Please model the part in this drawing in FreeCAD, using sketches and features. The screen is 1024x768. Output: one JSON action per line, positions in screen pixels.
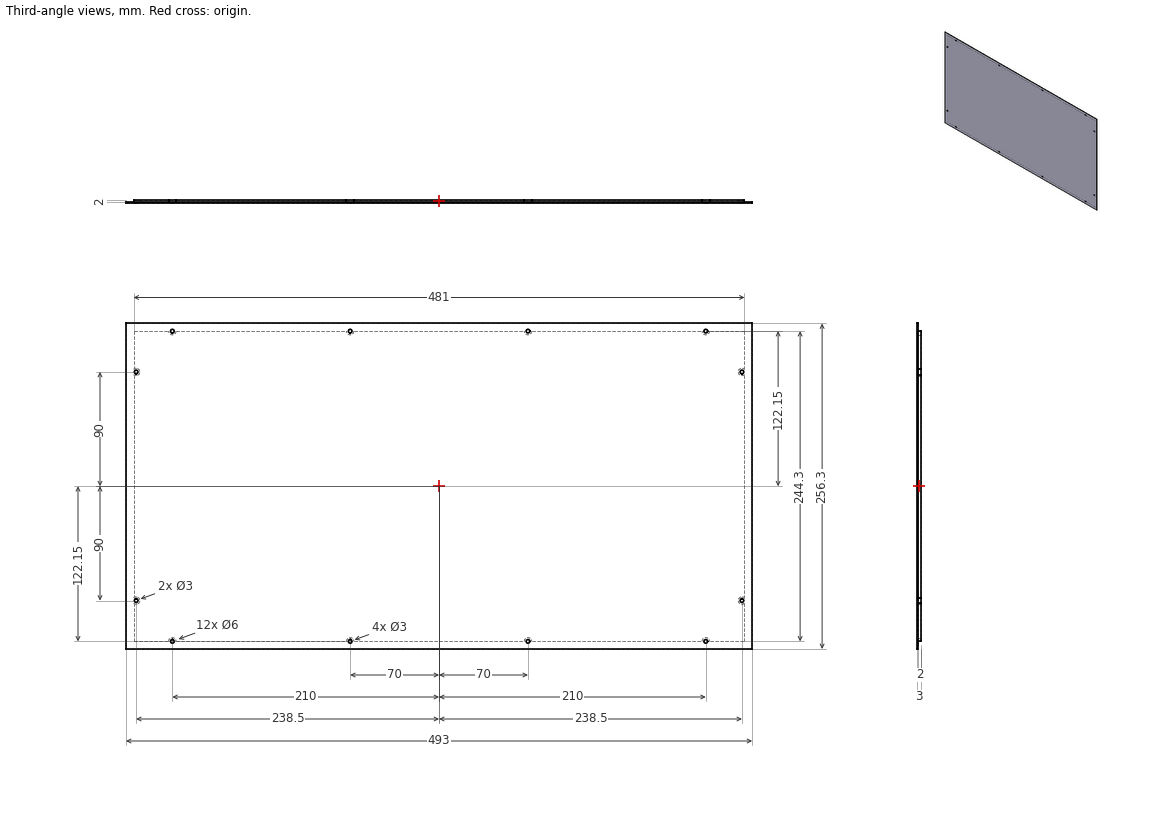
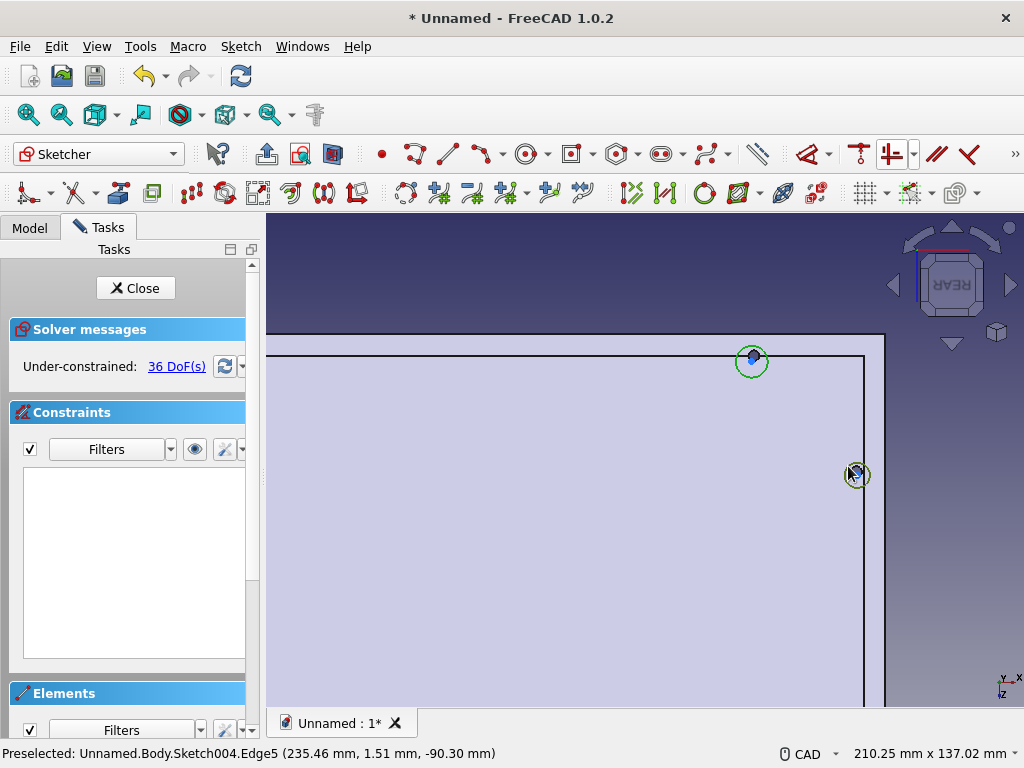
{"action": "scroll", "coordinate": [766, 350], "scroll_direction": "down", "scroll_amount": 7}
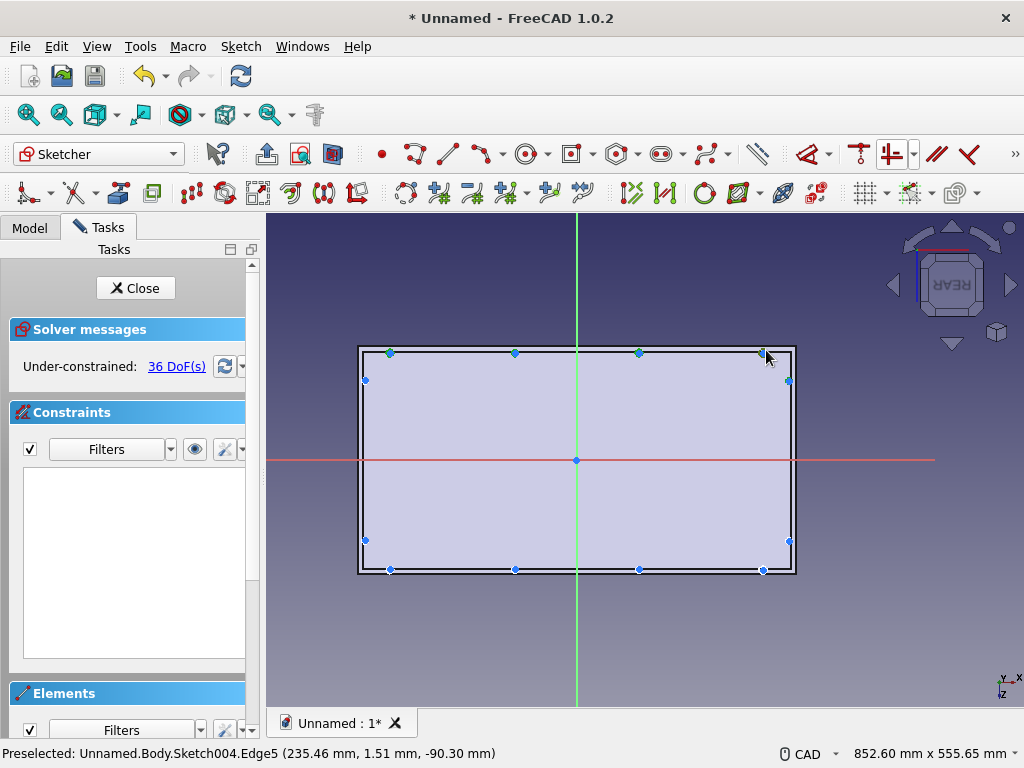
{"action": "scroll", "coordinate": [791, 539], "scroll_direction": "up", "scroll_amount": 8}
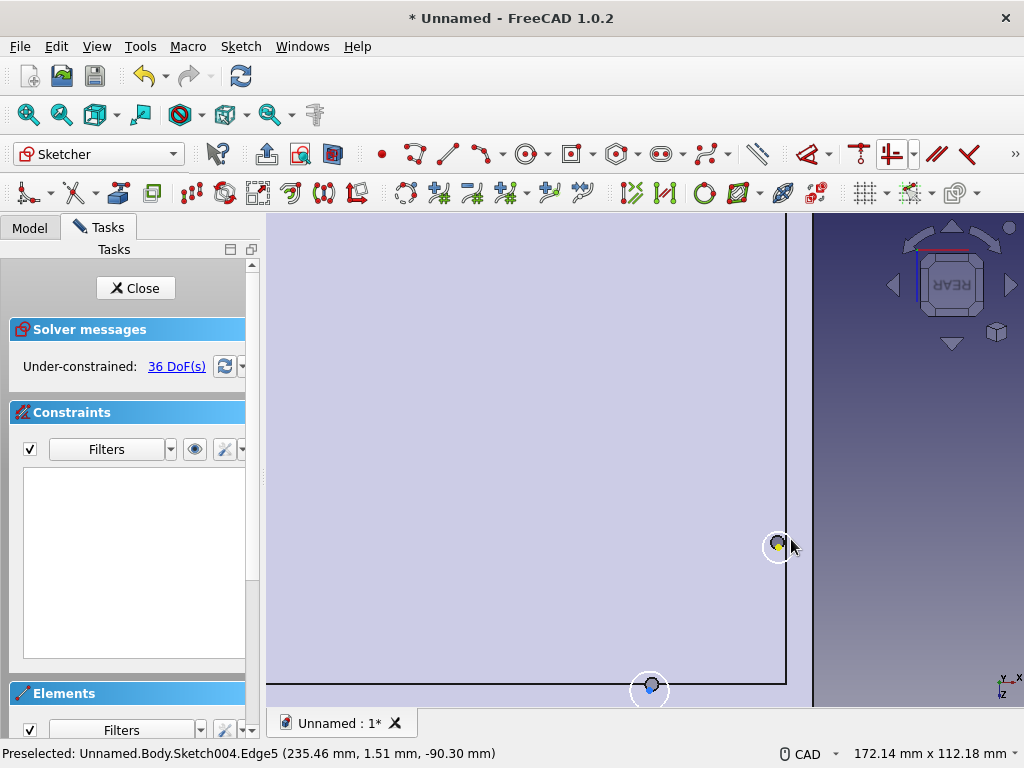
{"action": "left_click", "coordinate": [789, 536]}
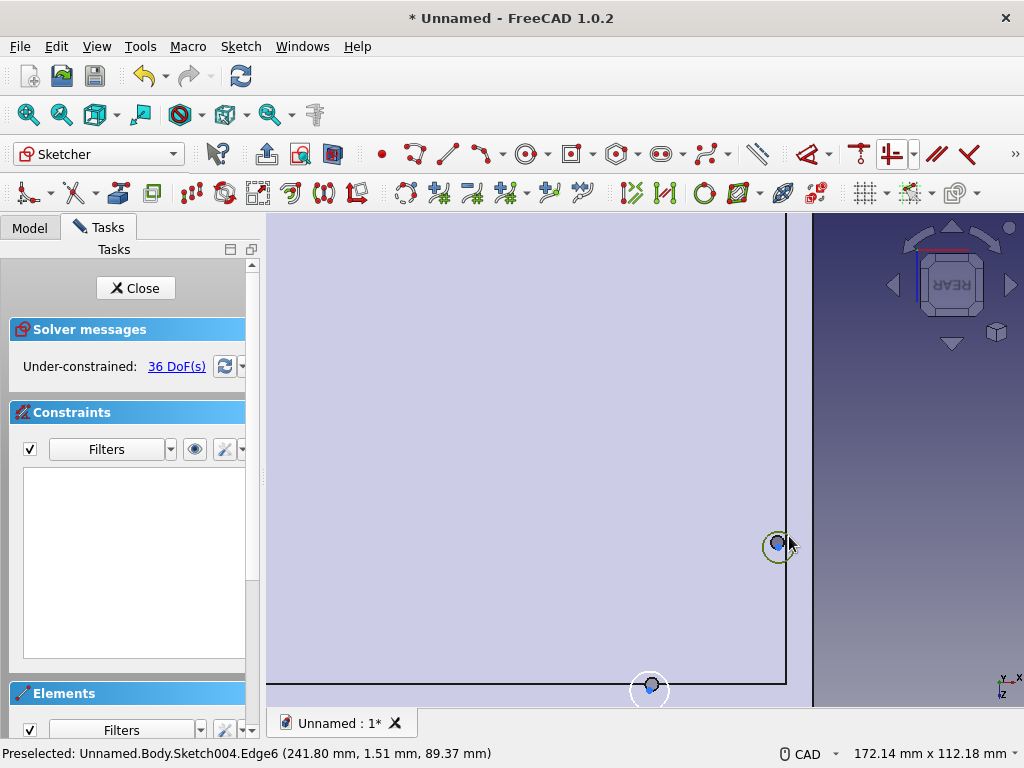
{"action": "left_click", "coordinate": [663, 677]}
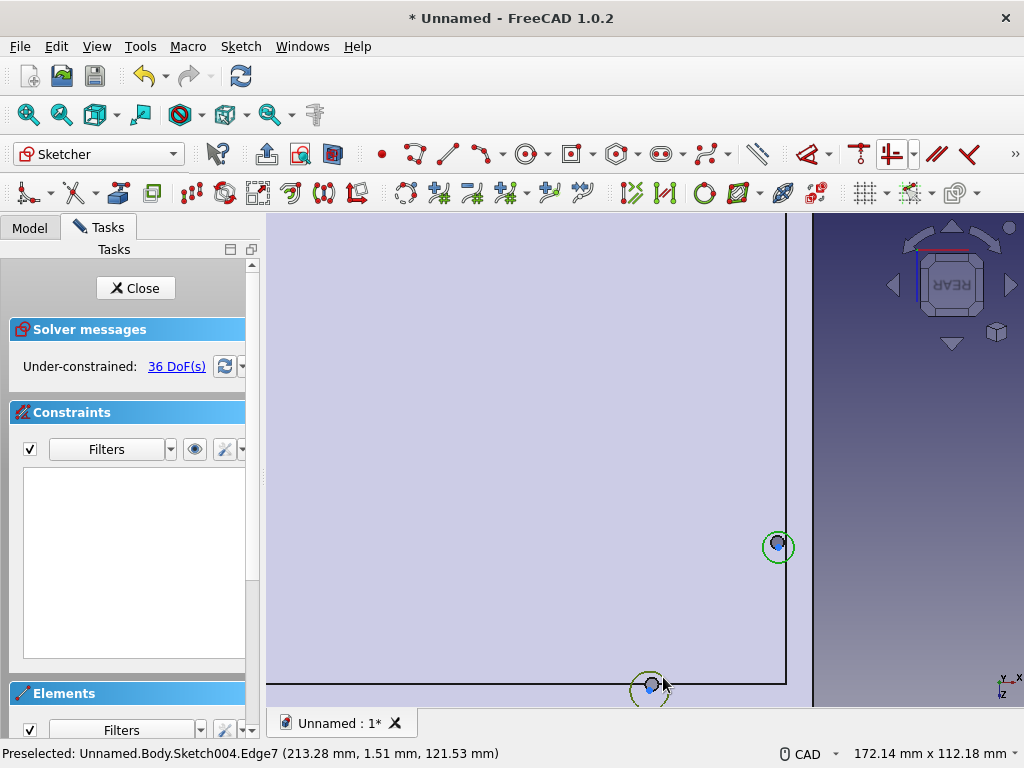
{"action": "scroll", "coordinate": [791, 539], "scroll_direction": "down", "scroll_amount": 8}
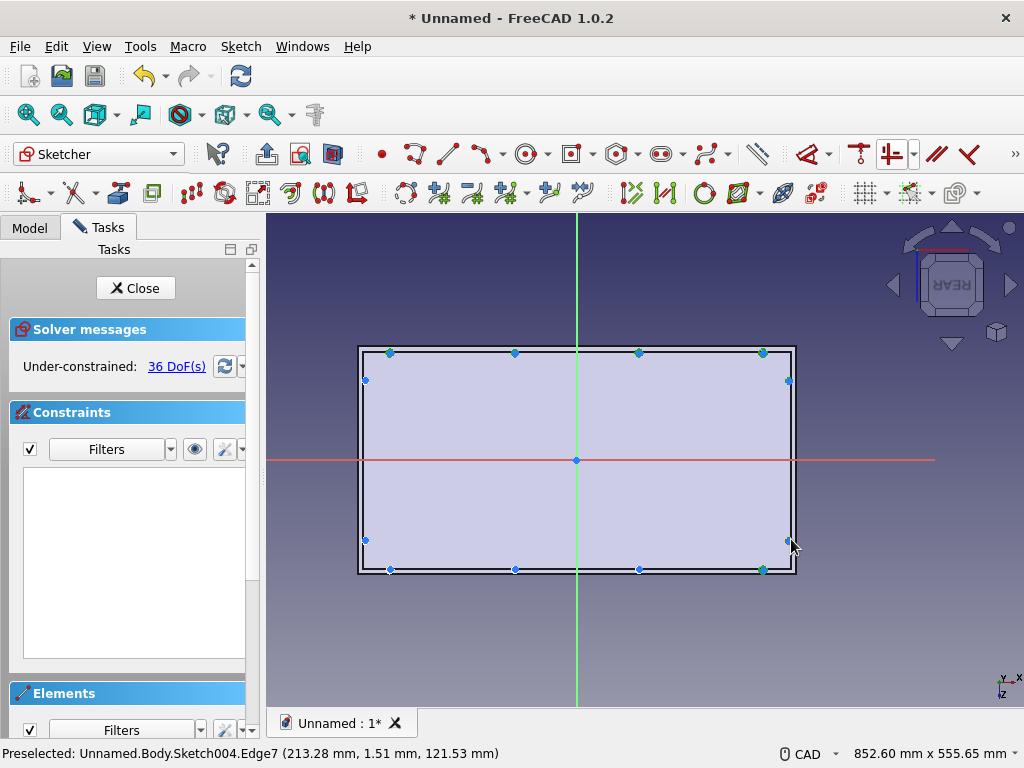
{"action": "scroll", "coordinate": [641, 568], "scroll_direction": "up", "scroll_amount": 7}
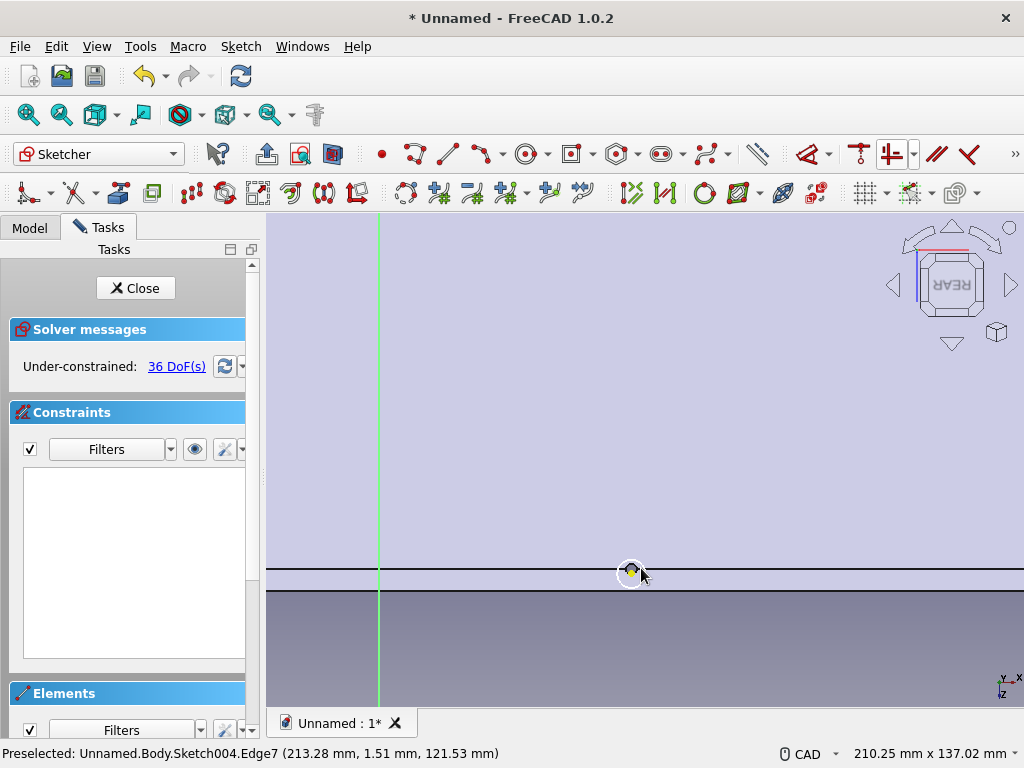
{"action": "left_click", "coordinate": [641, 564]}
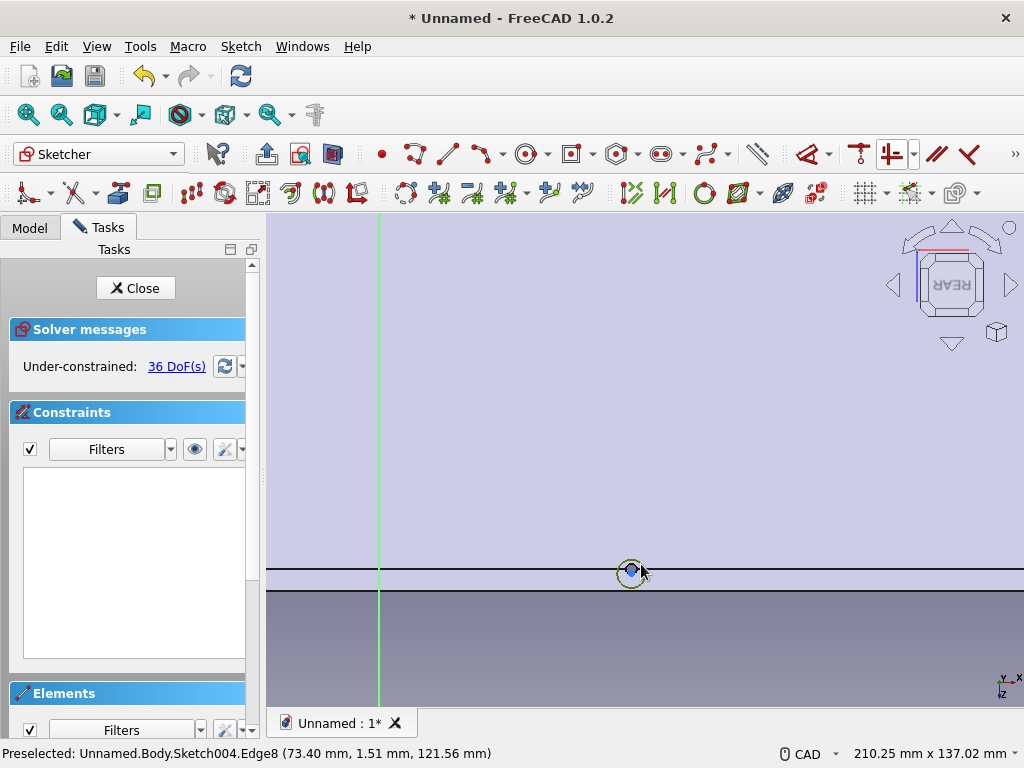
{"action": "scroll", "coordinate": [641, 568], "scroll_direction": "down", "scroll_amount": 7}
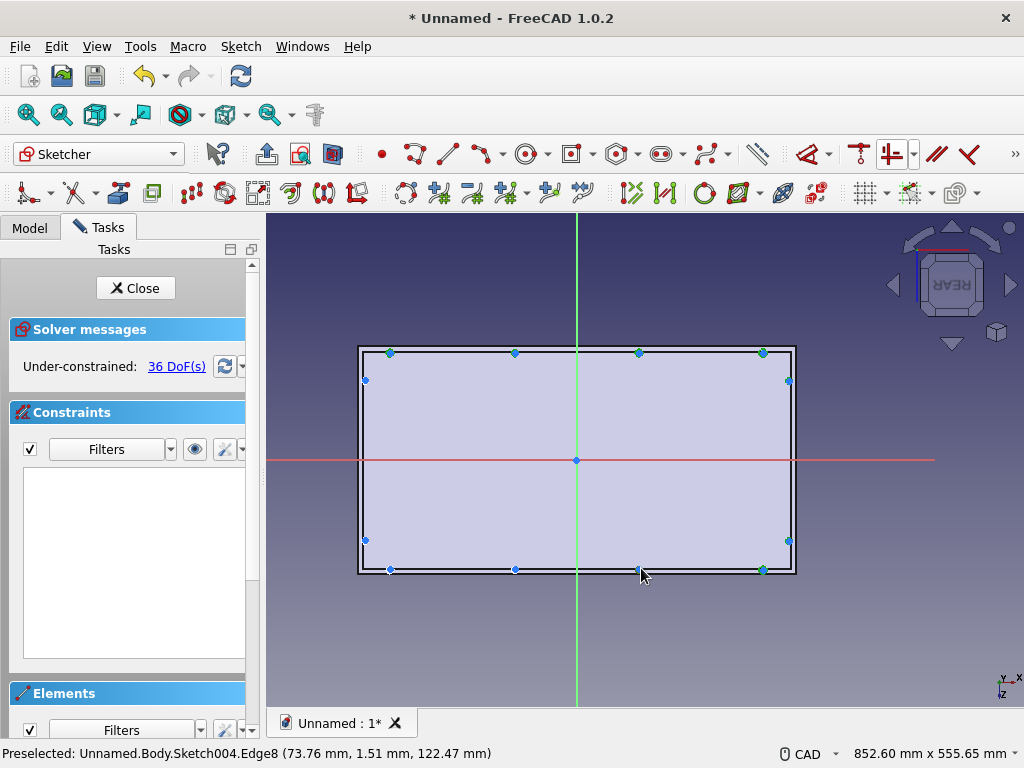
{"action": "scroll", "coordinate": [517, 568], "scroll_direction": "up", "scroll_amount": 8}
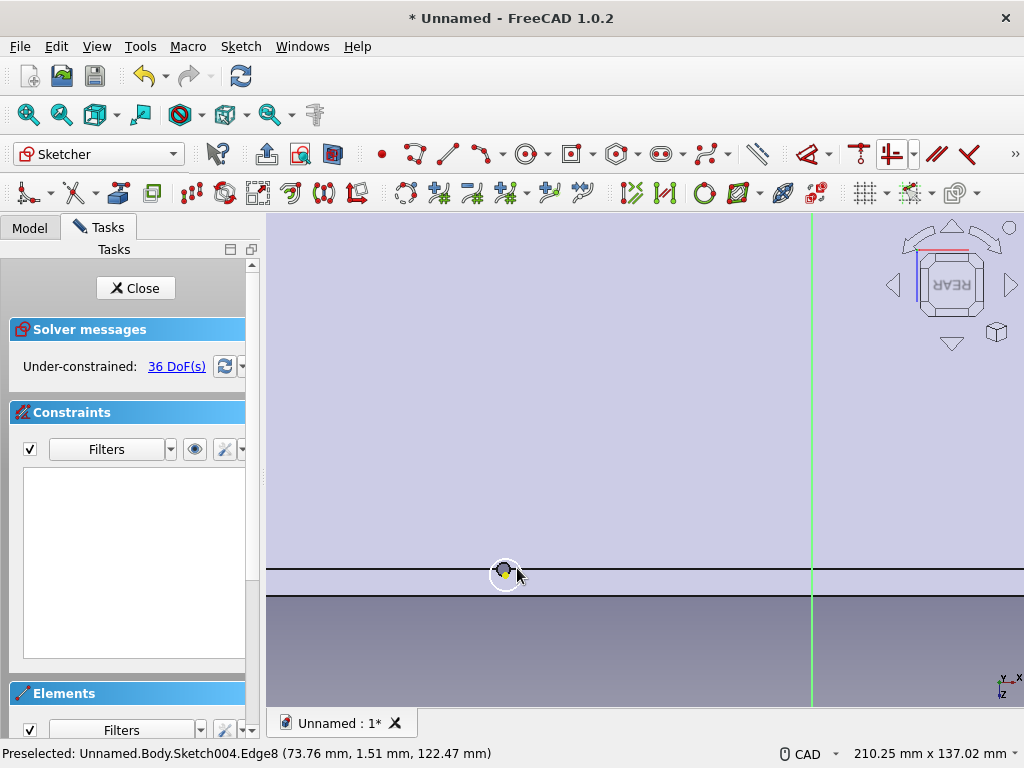
{"action": "left_click", "coordinate": [517, 564]}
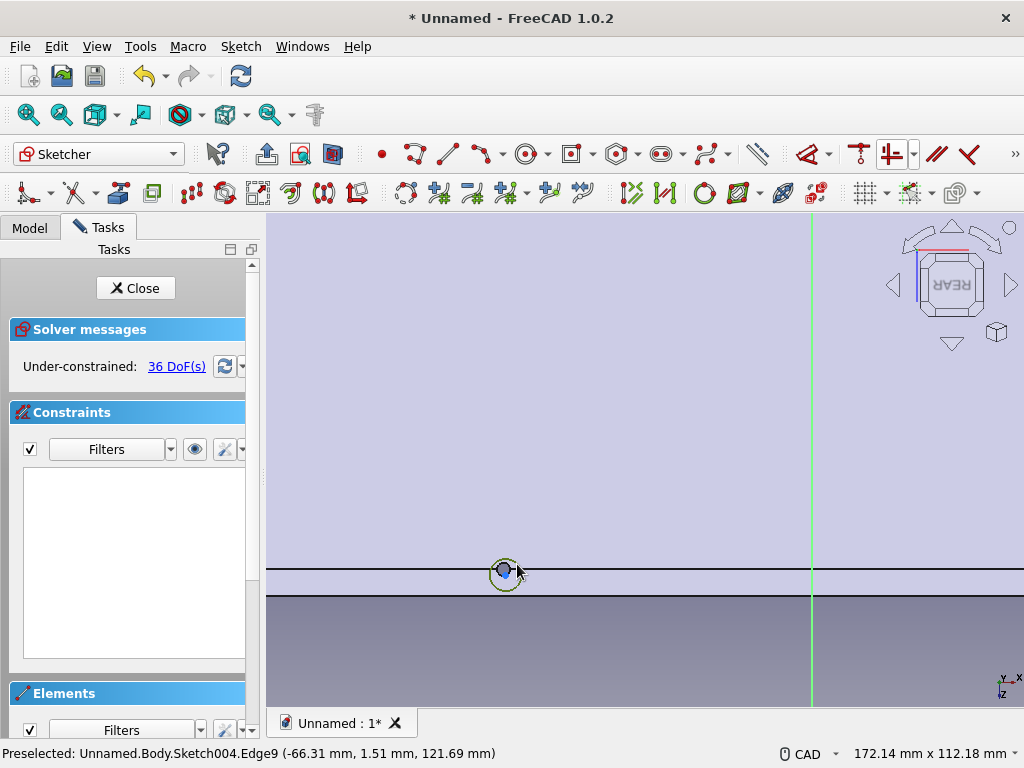
{"action": "scroll", "coordinate": [517, 568], "scroll_direction": "down", "scroll_amount": 8}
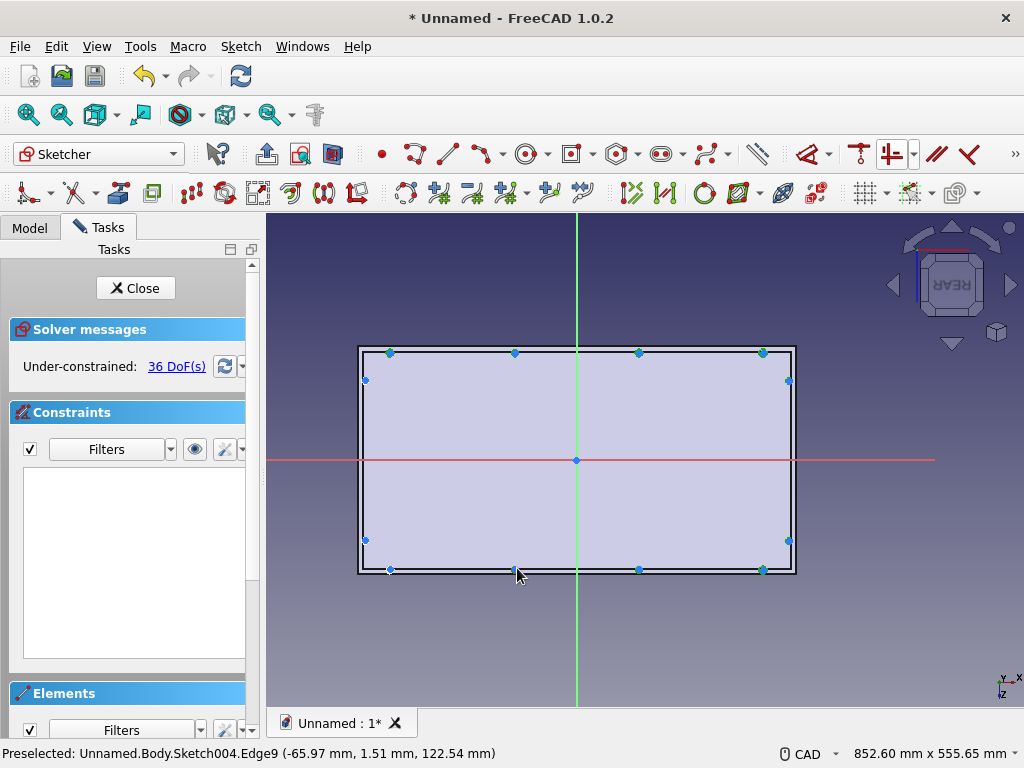
{"action": "scroll", "coordinate": [392, 568], "scroll_direction": "up", "scroll_amount": 7}